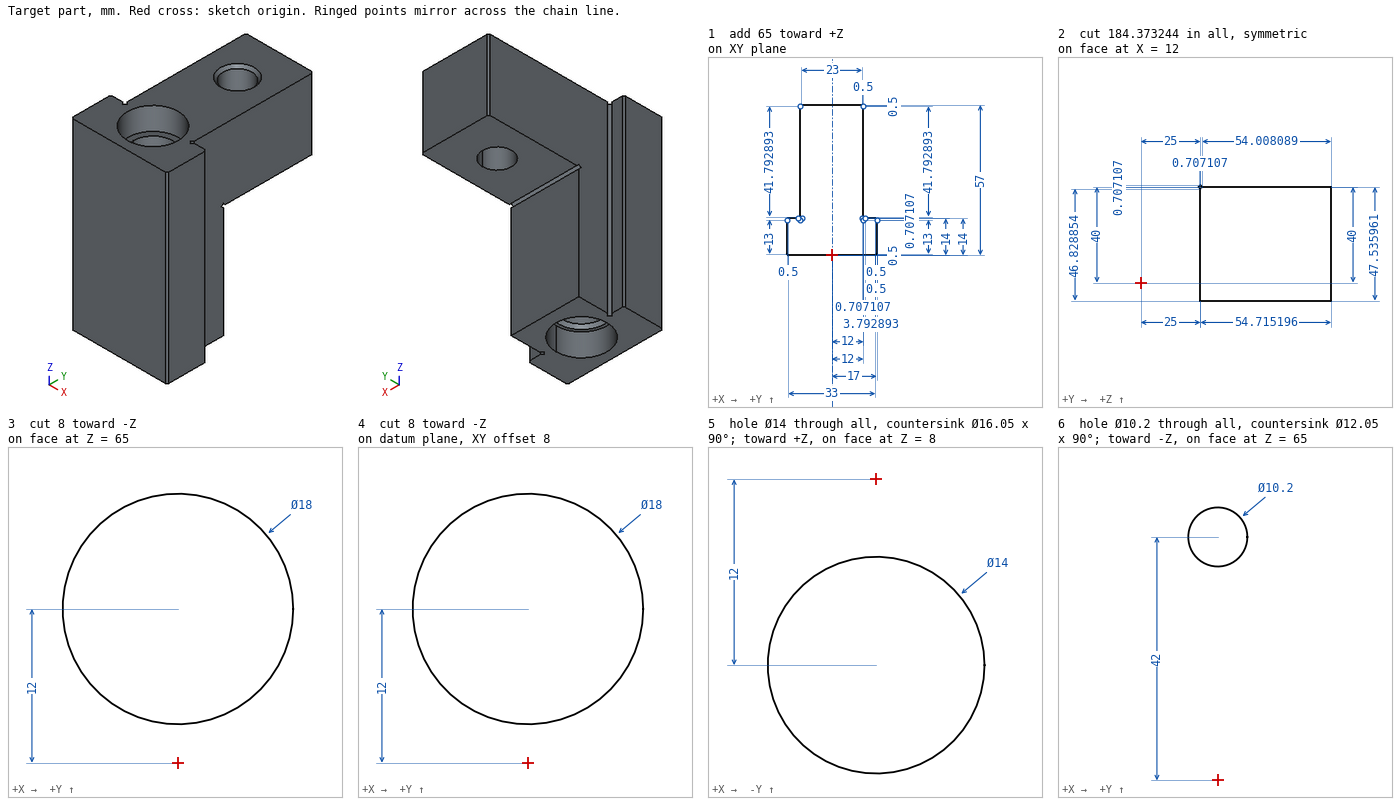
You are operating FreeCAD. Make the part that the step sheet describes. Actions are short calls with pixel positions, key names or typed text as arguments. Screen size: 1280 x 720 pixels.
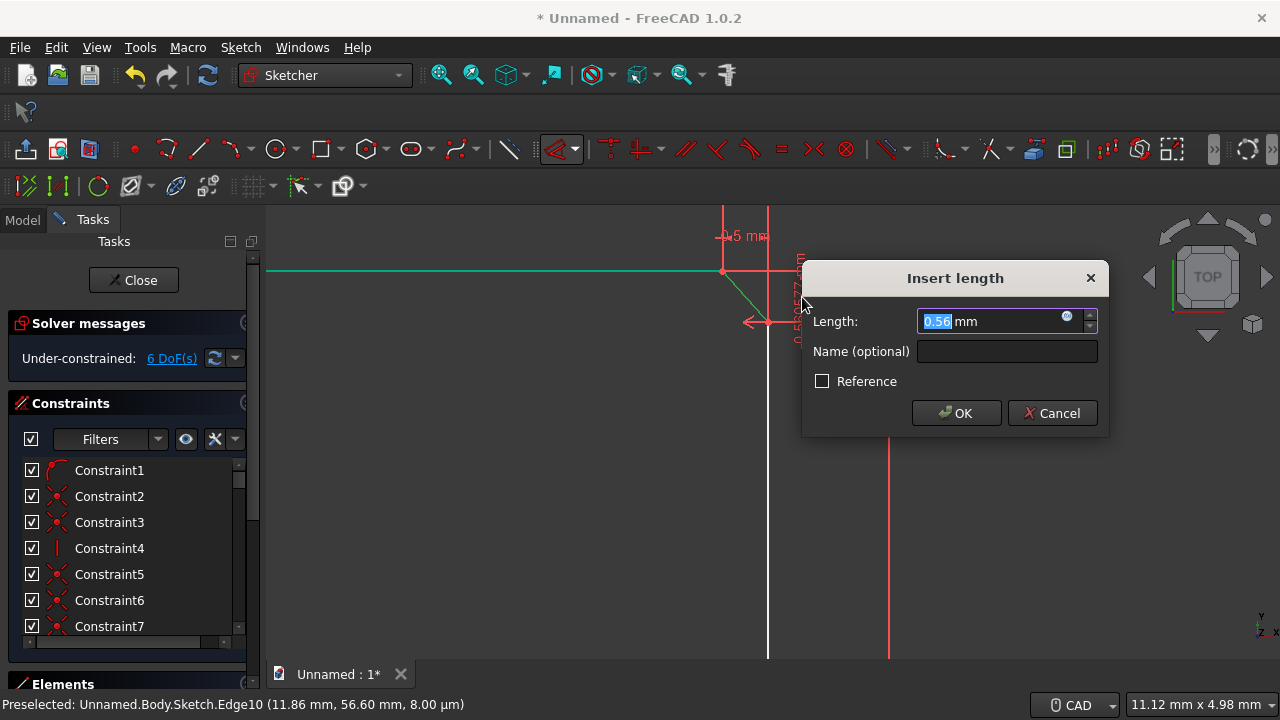
text(0.5)
key(Return)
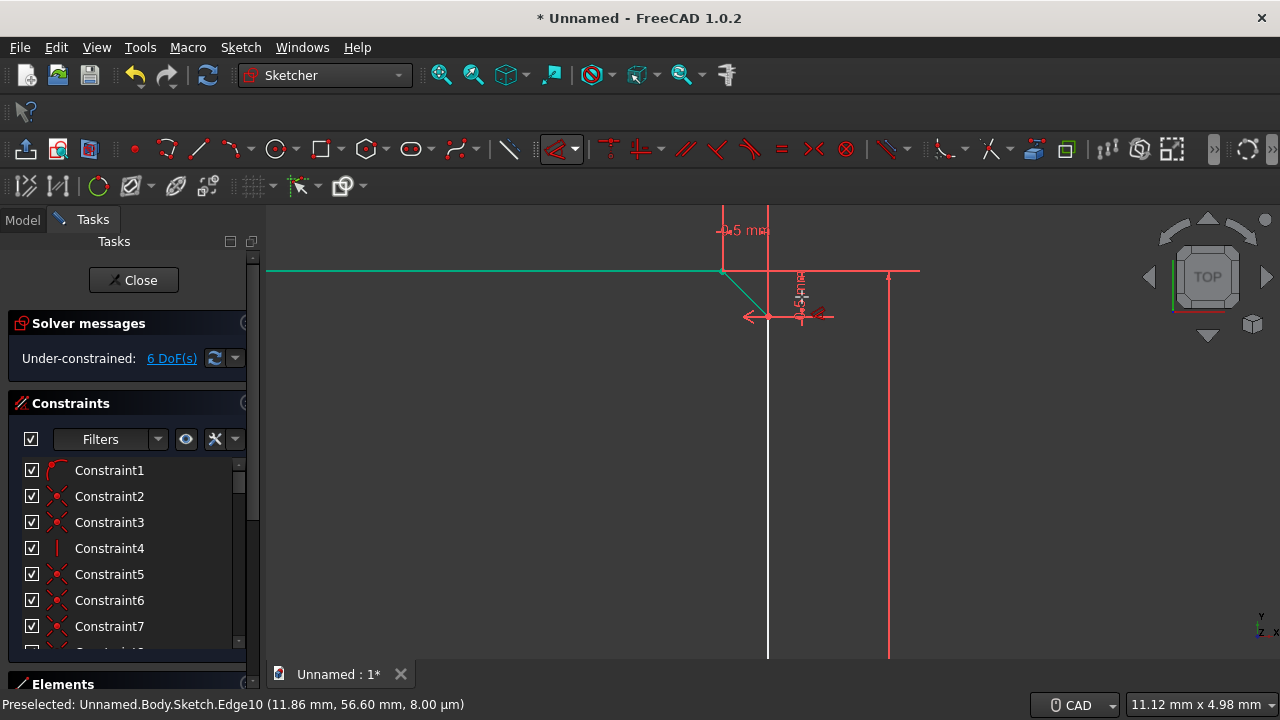
scroll(758, 304, down, 15)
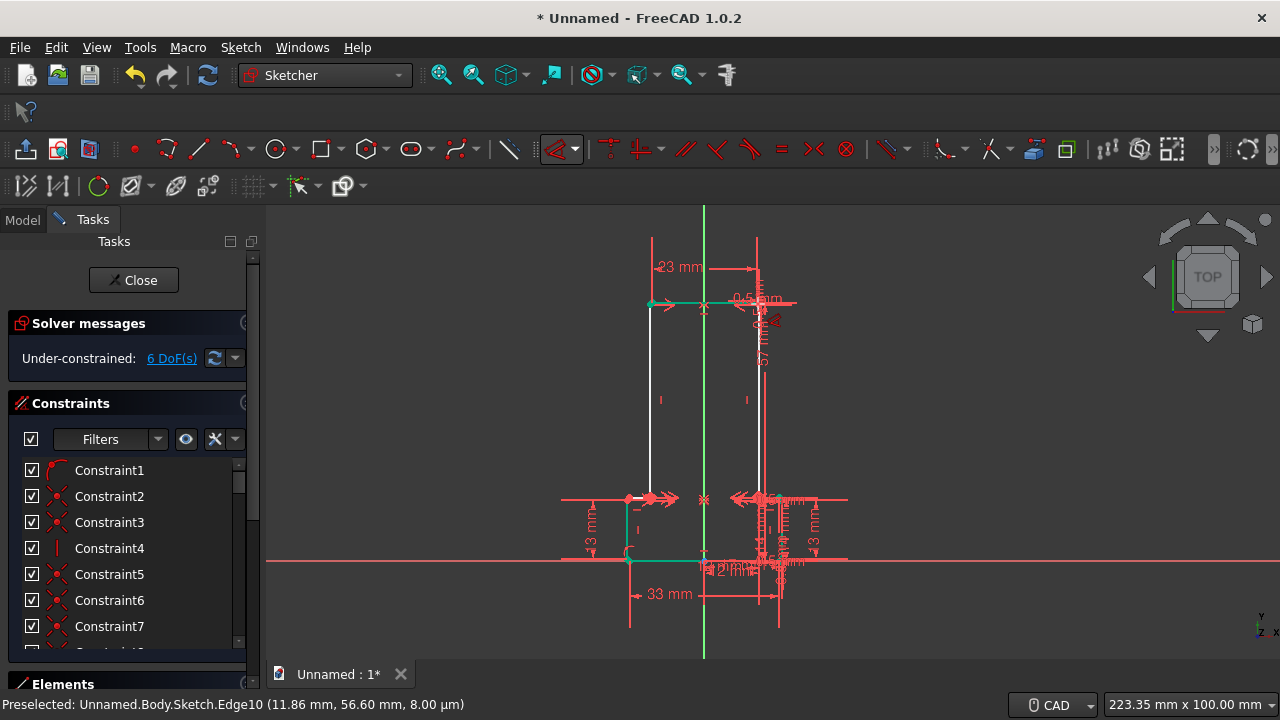
scroll(629, 498, up, 15)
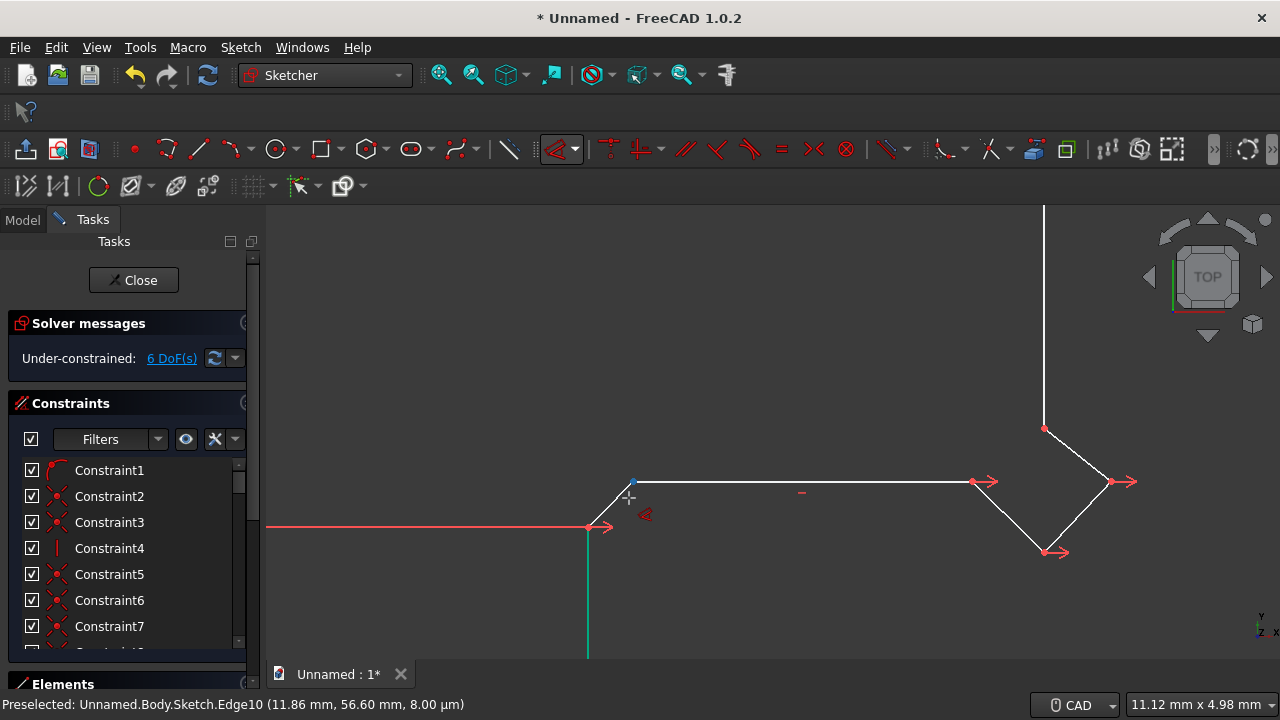
click(620, 495)
click(611, 561)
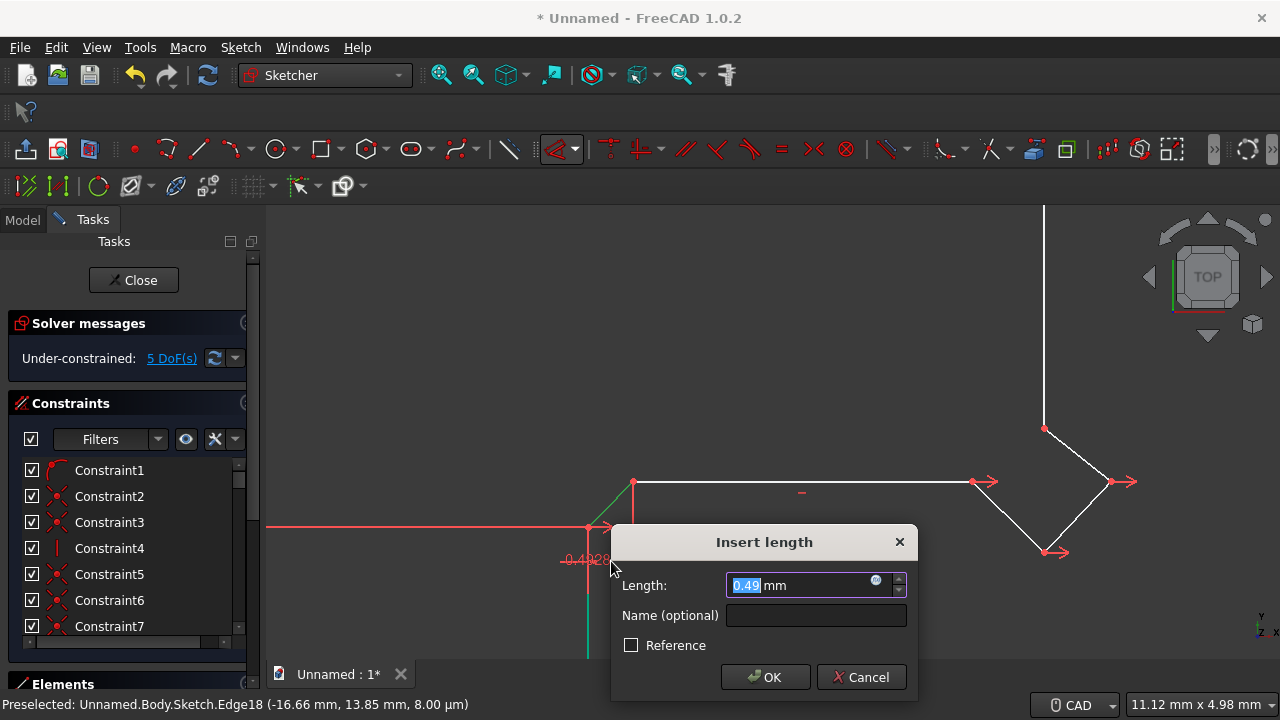
text(0.5)
key(Return)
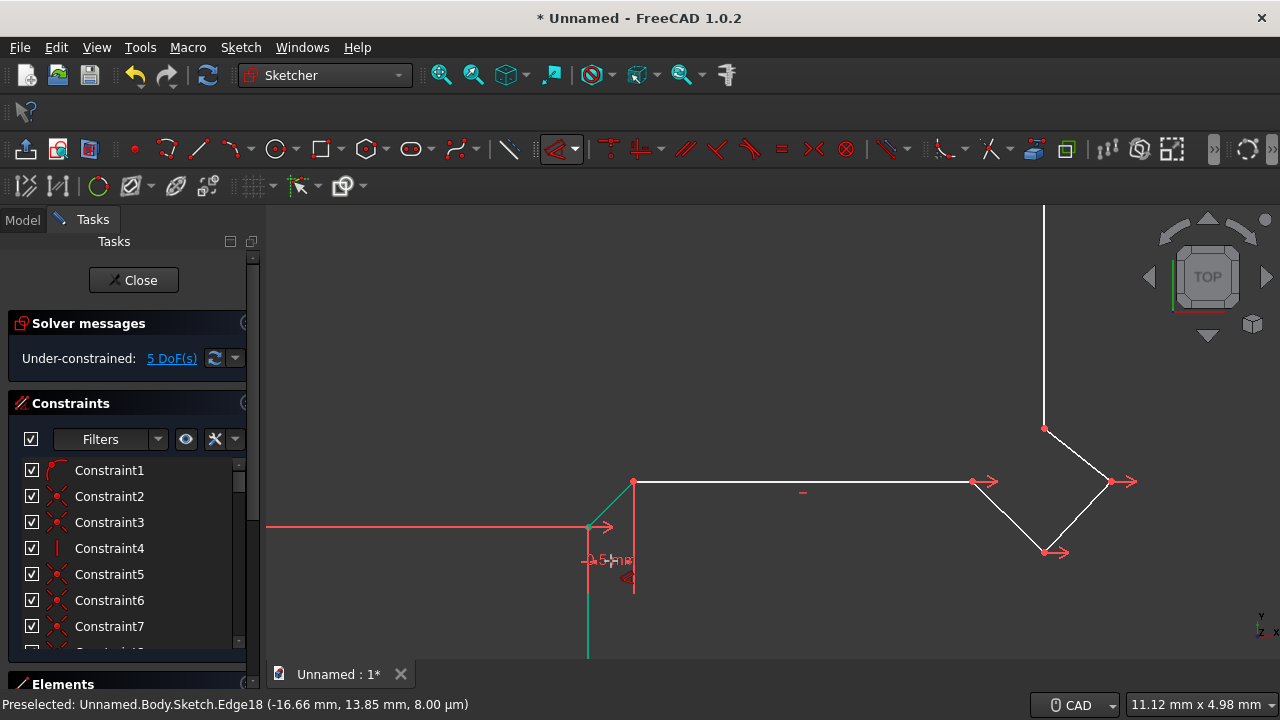
scroll(629, 499, down, 15)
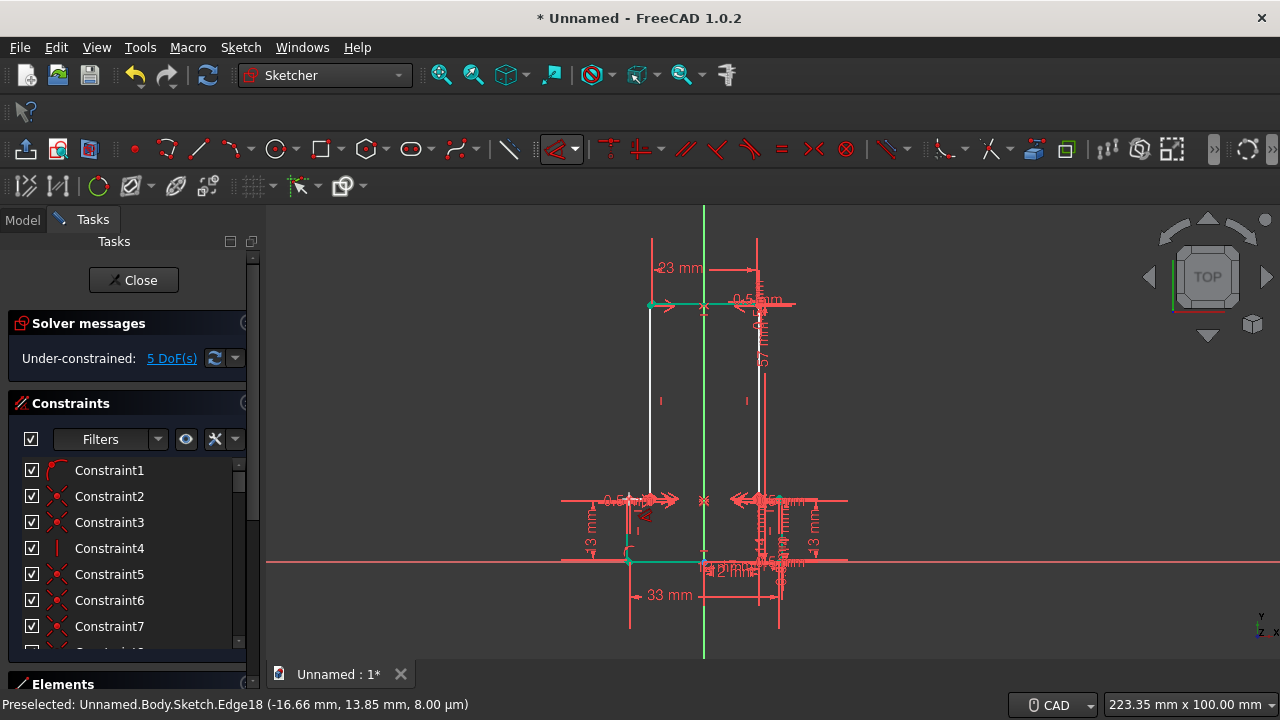
scroll(774, 499, up, 6)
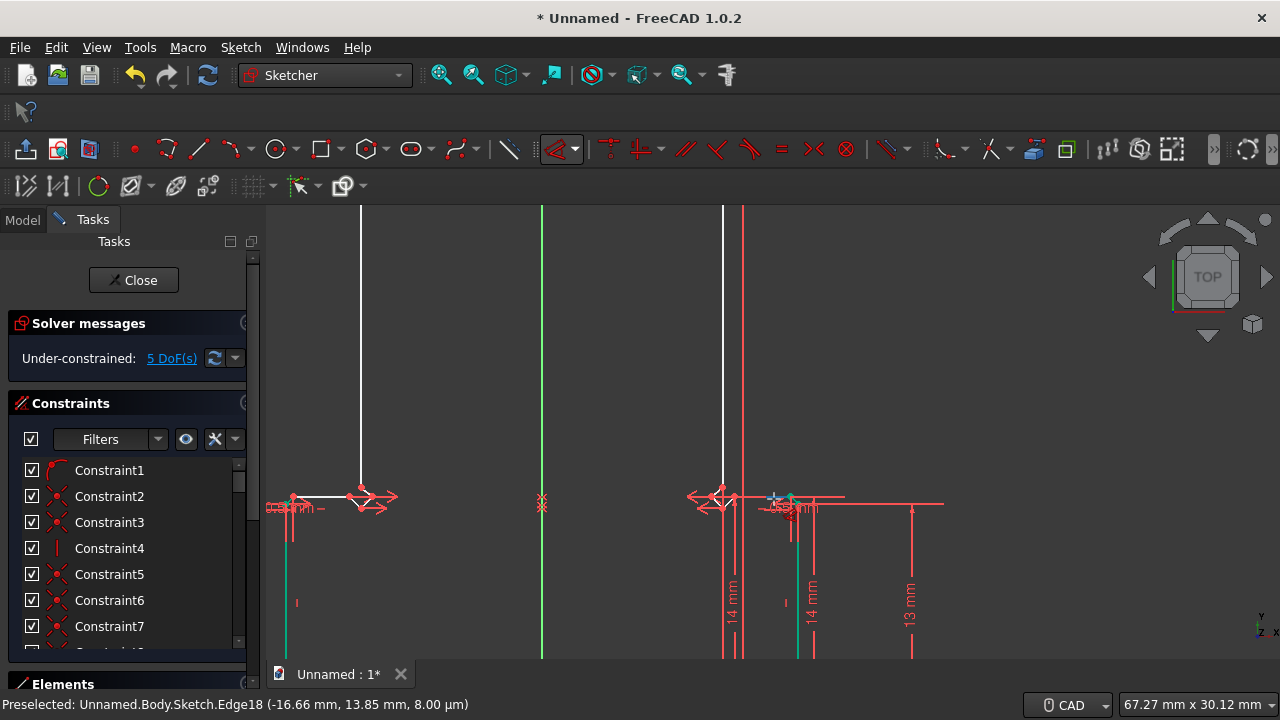
click(774, 497)
click(763, 531)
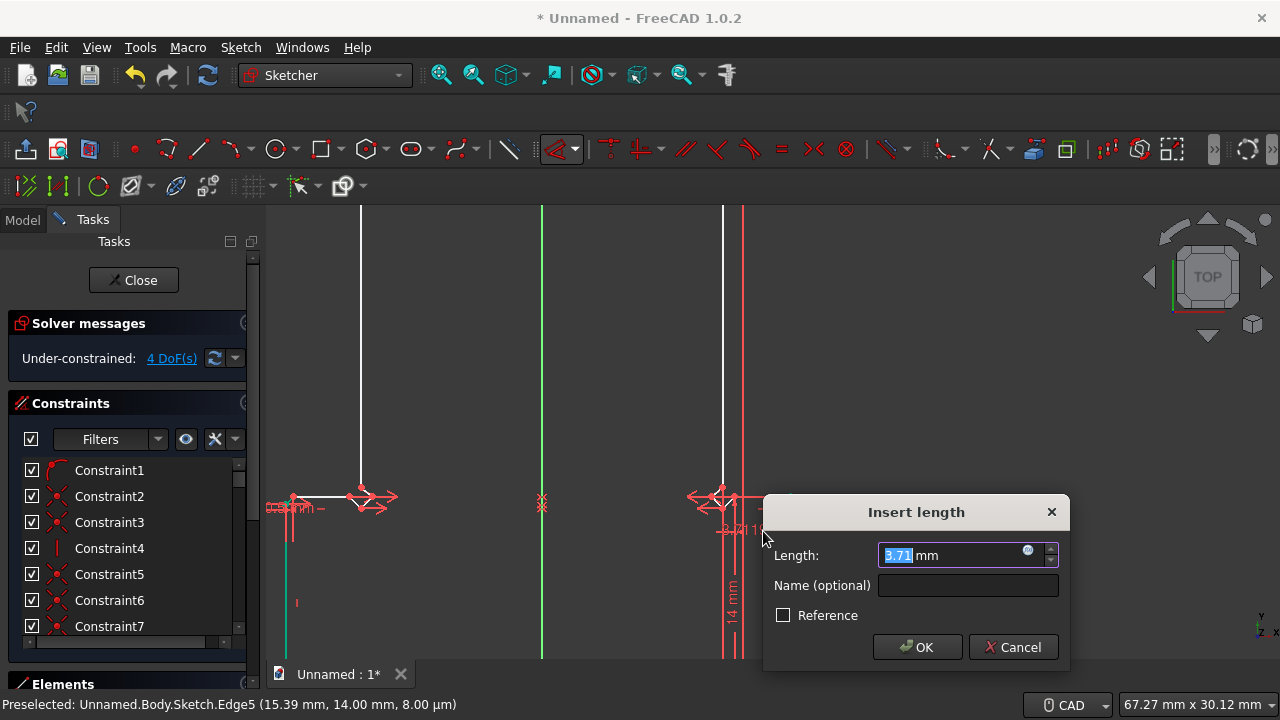
text(3.792893)
key(Return)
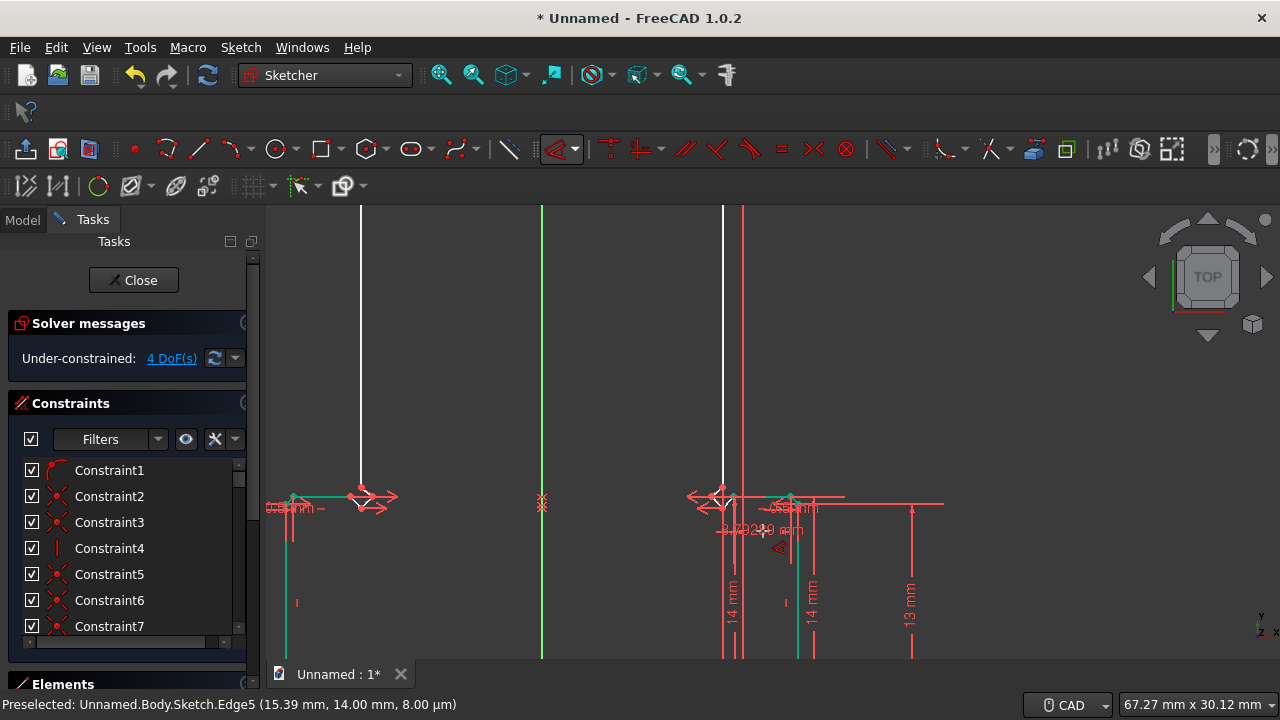
click(723, 298)
click(757, 360)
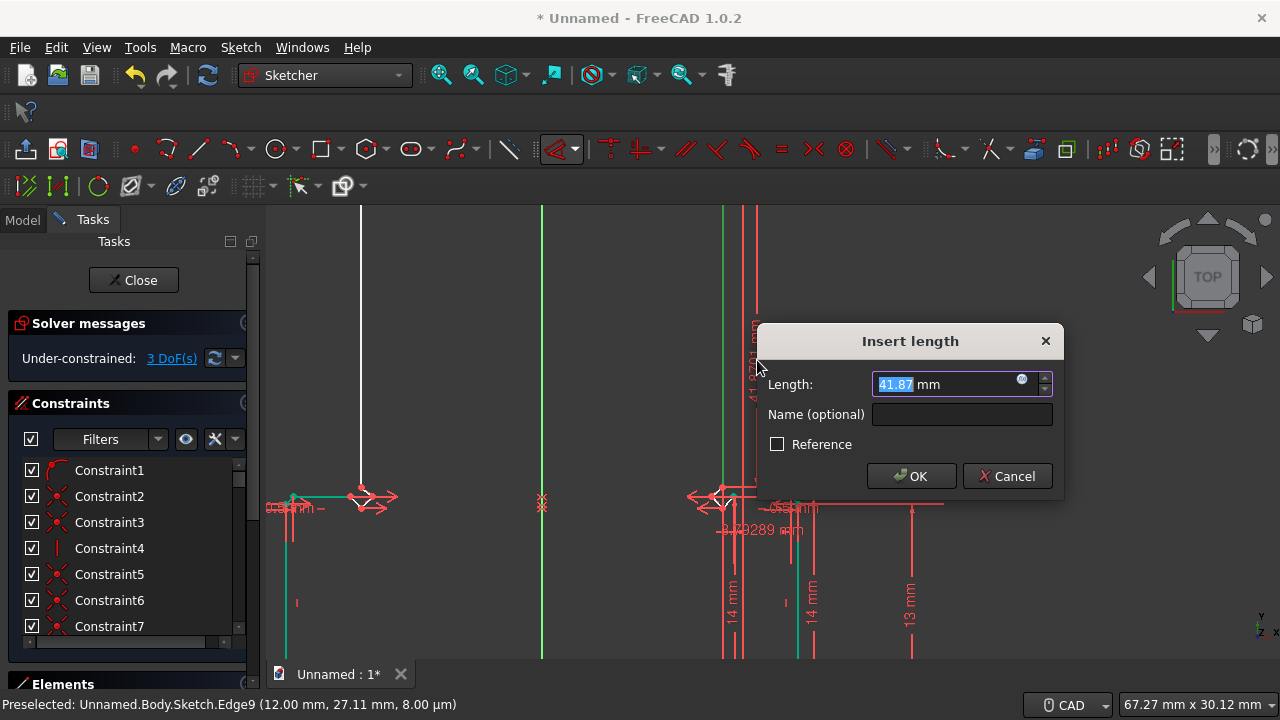
text(41.792893)
key(Return)